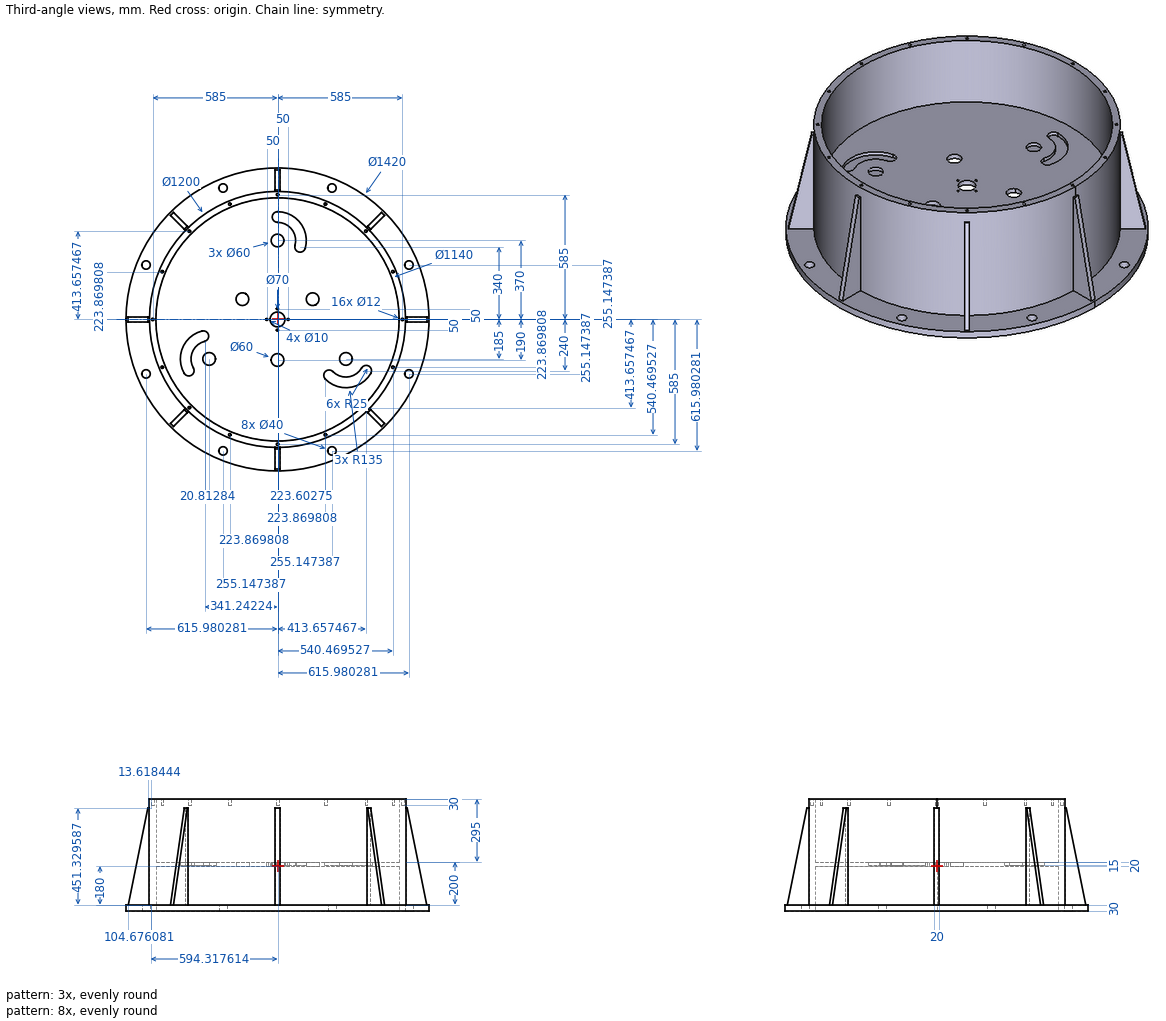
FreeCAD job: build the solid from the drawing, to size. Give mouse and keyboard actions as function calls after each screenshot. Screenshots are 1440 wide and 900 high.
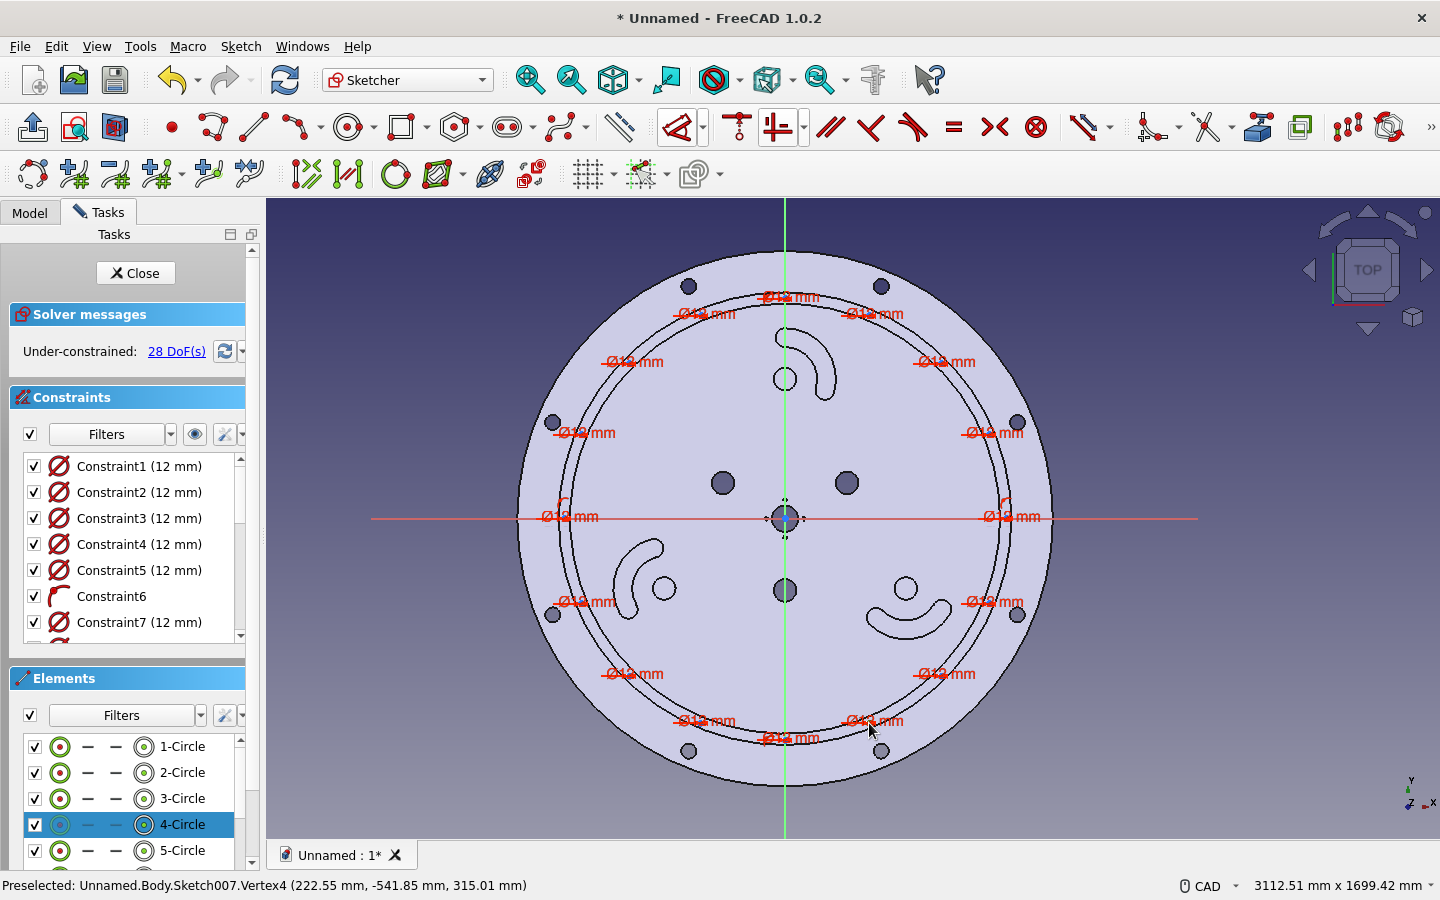
click(701, 723)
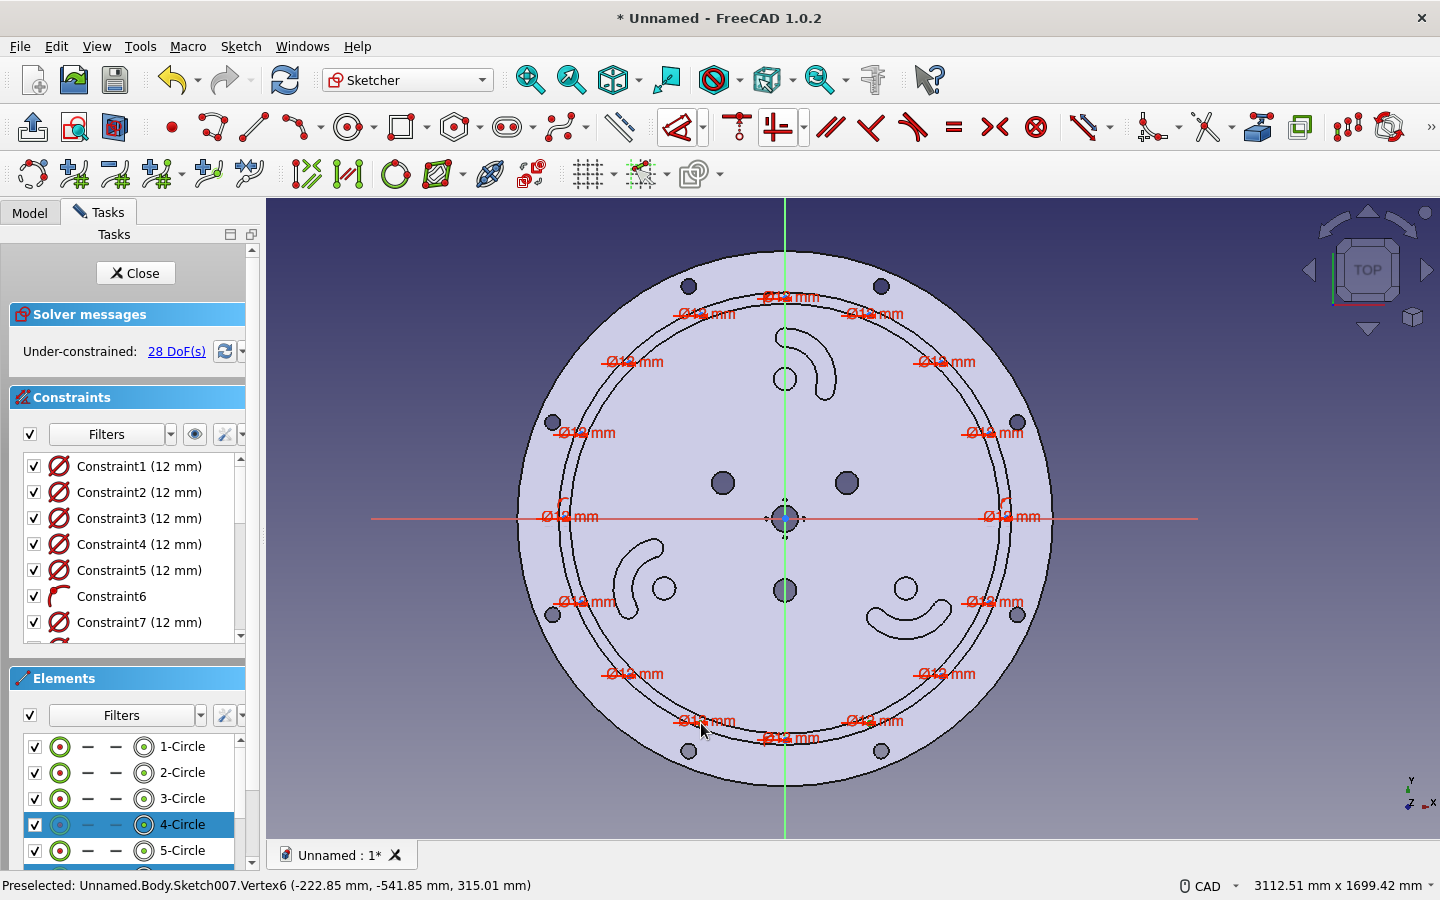
key(h)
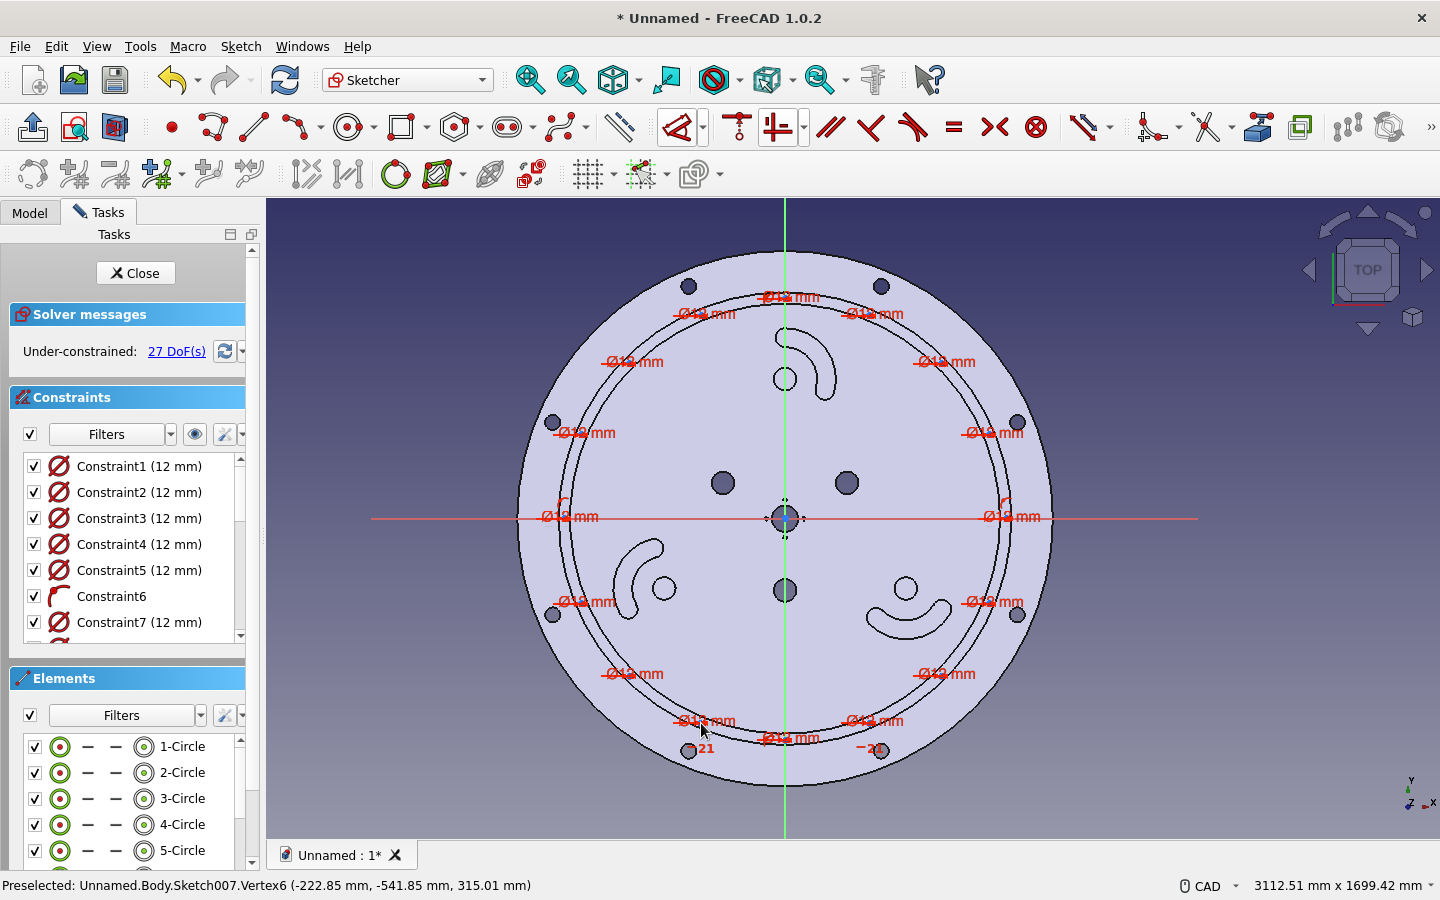
click(941, 676)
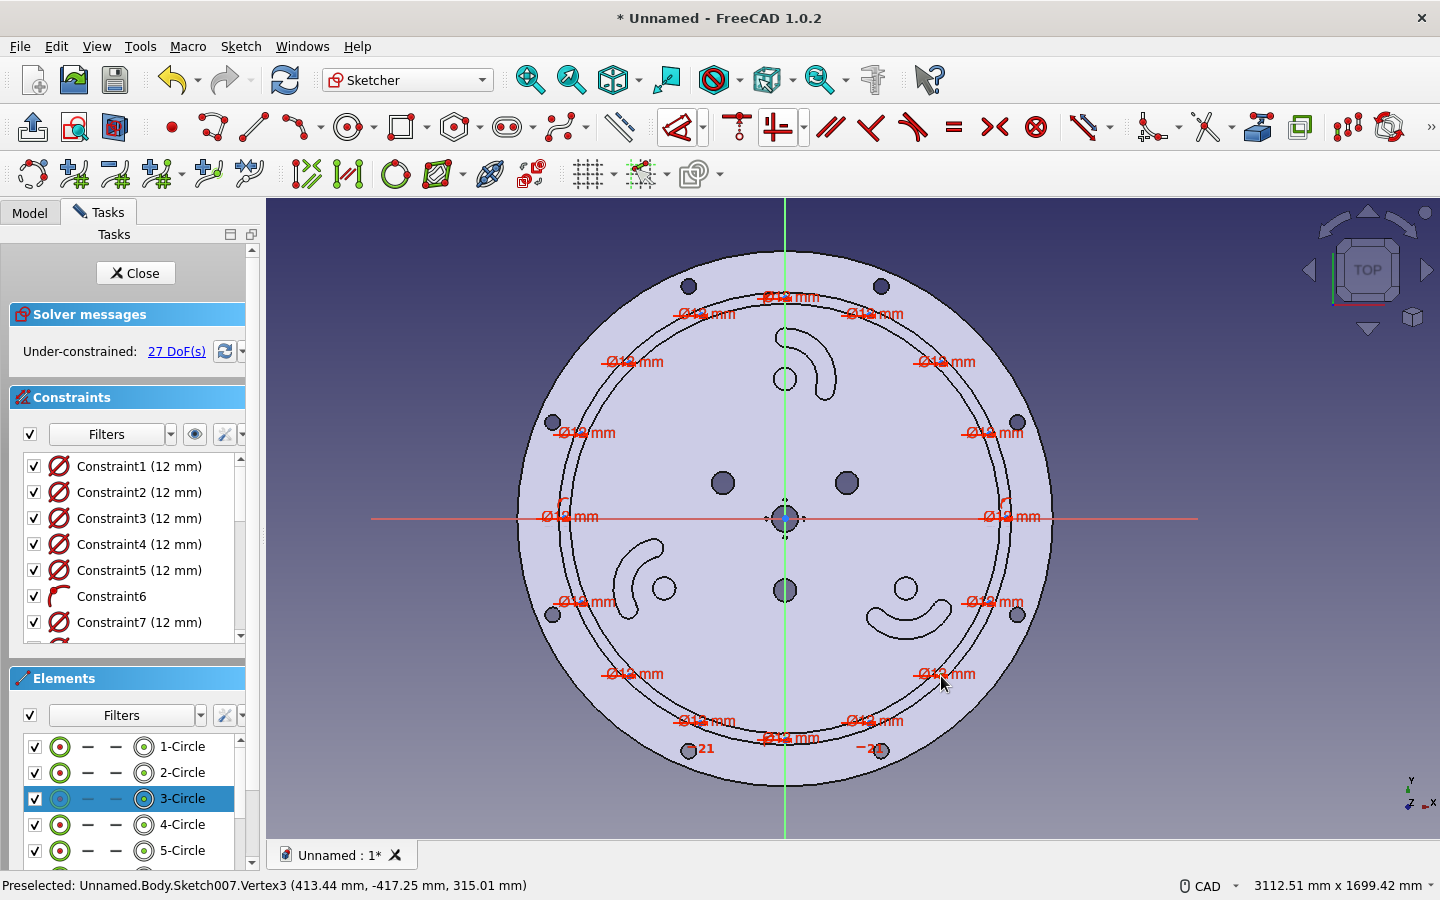
click(629, 676)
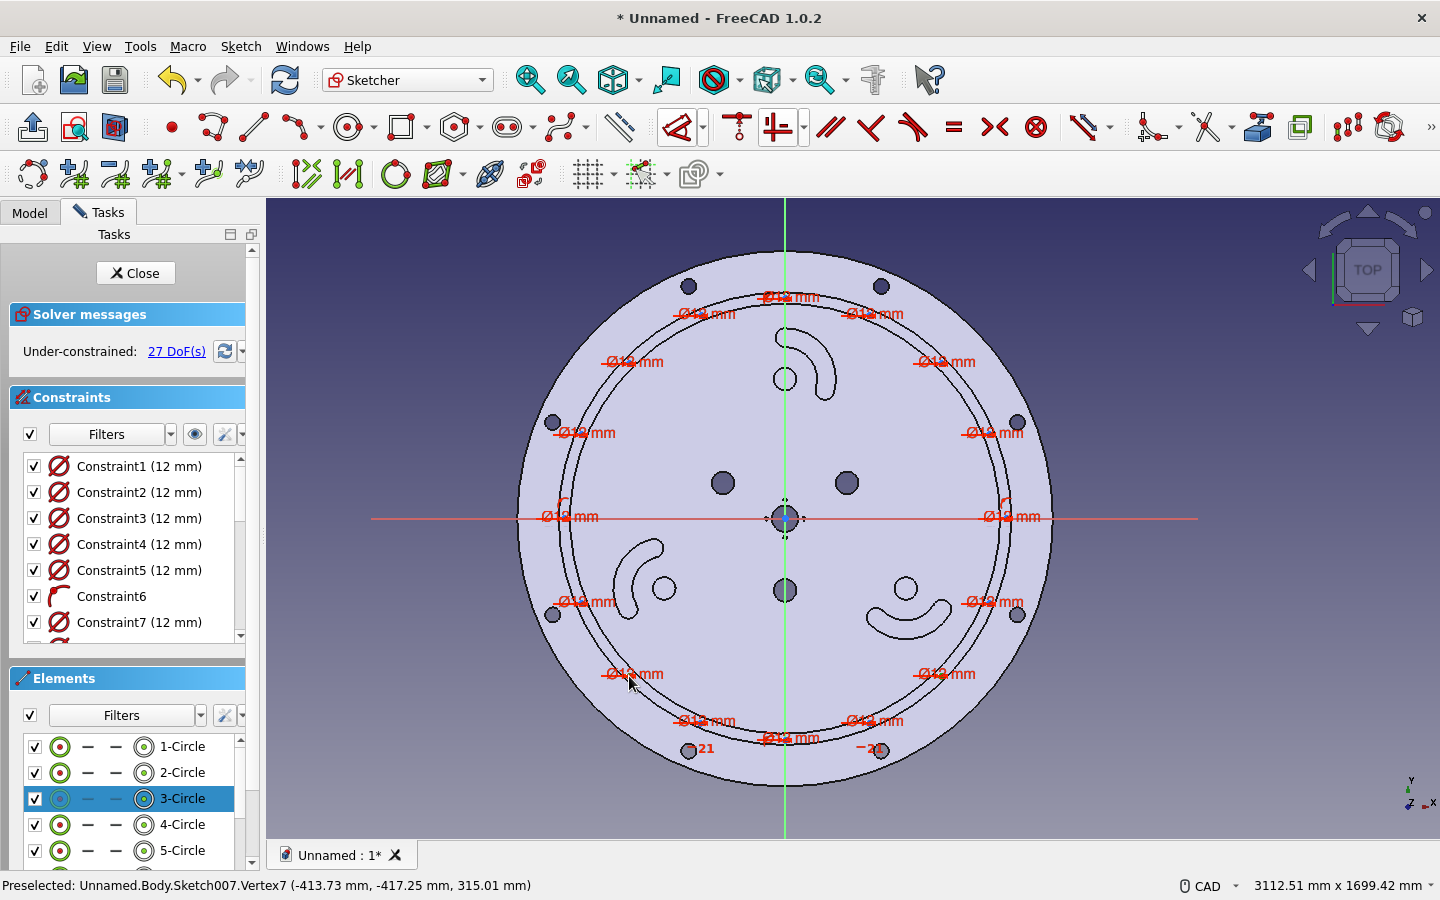
key(h)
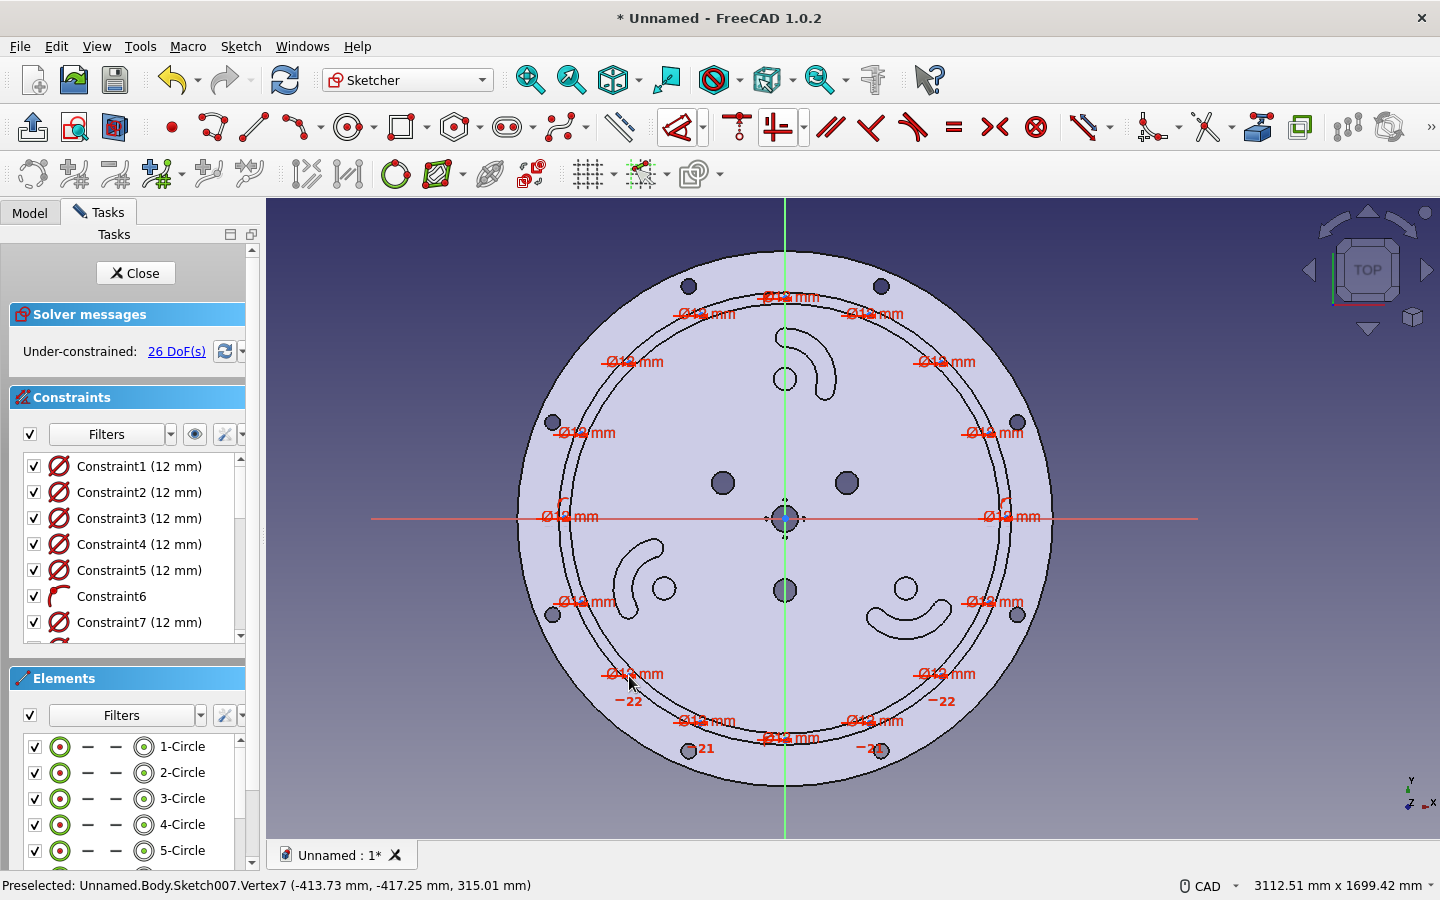
click(989, 604)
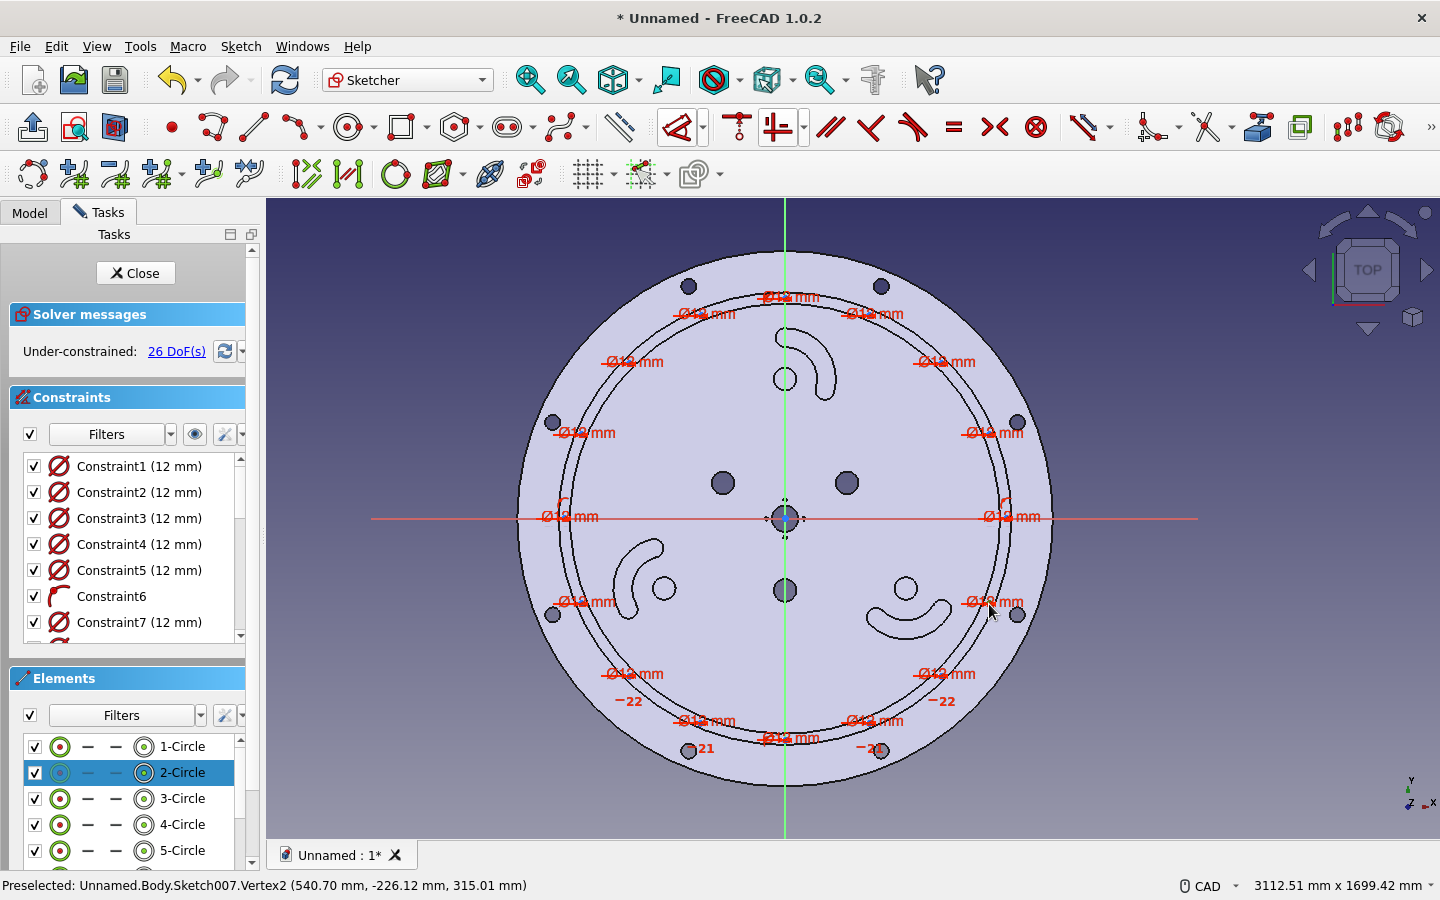
click(581, 604)